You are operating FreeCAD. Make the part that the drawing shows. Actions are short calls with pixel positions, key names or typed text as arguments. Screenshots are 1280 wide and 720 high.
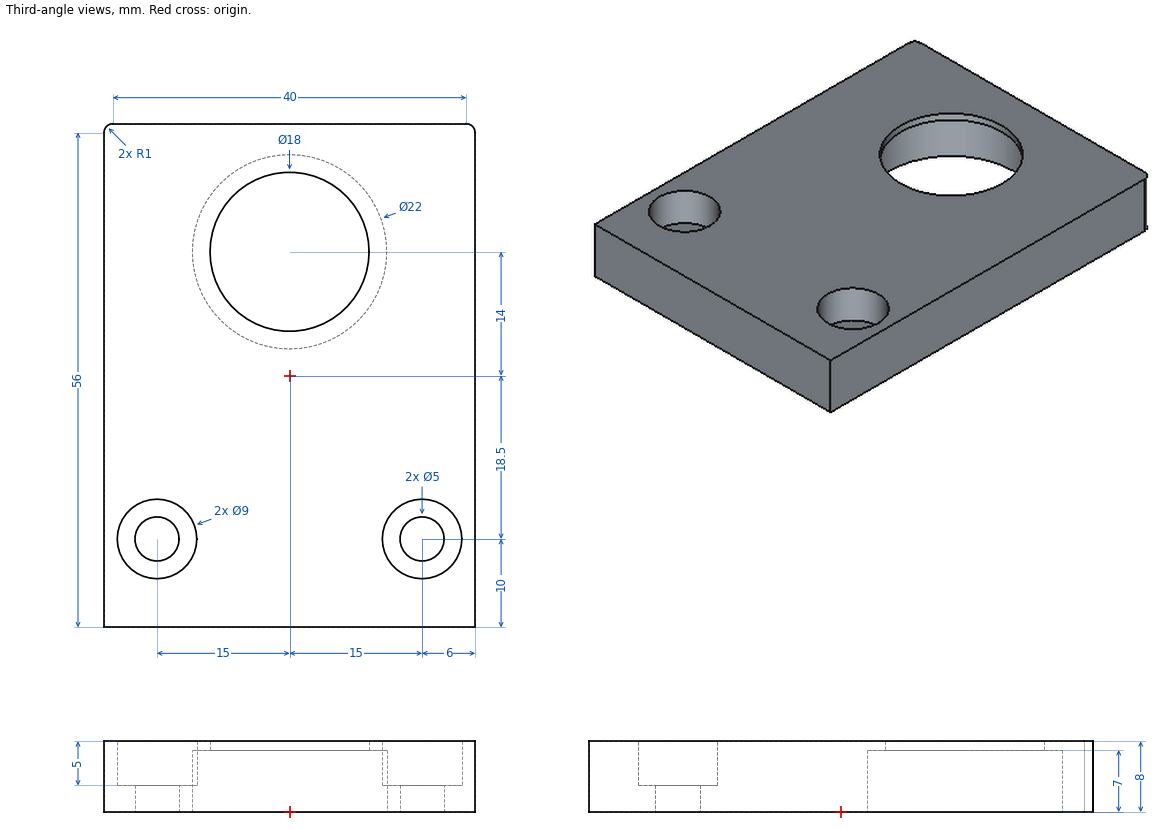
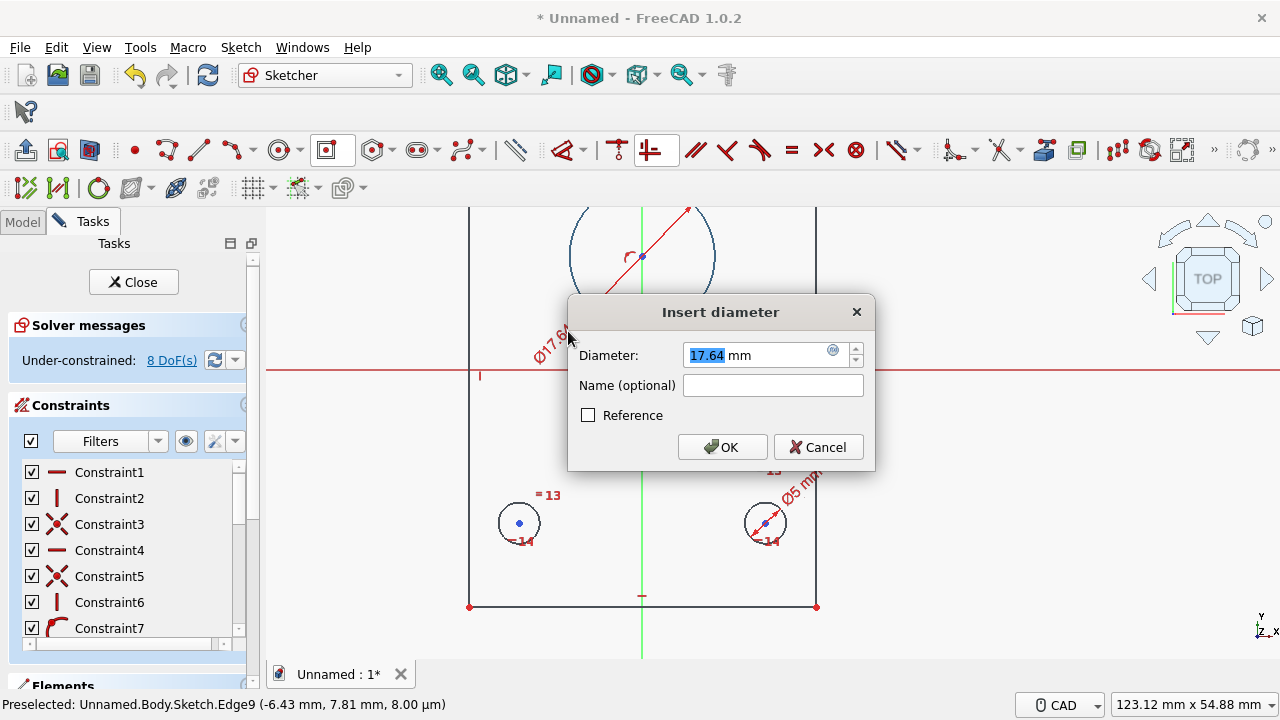
text(18)
key(Return)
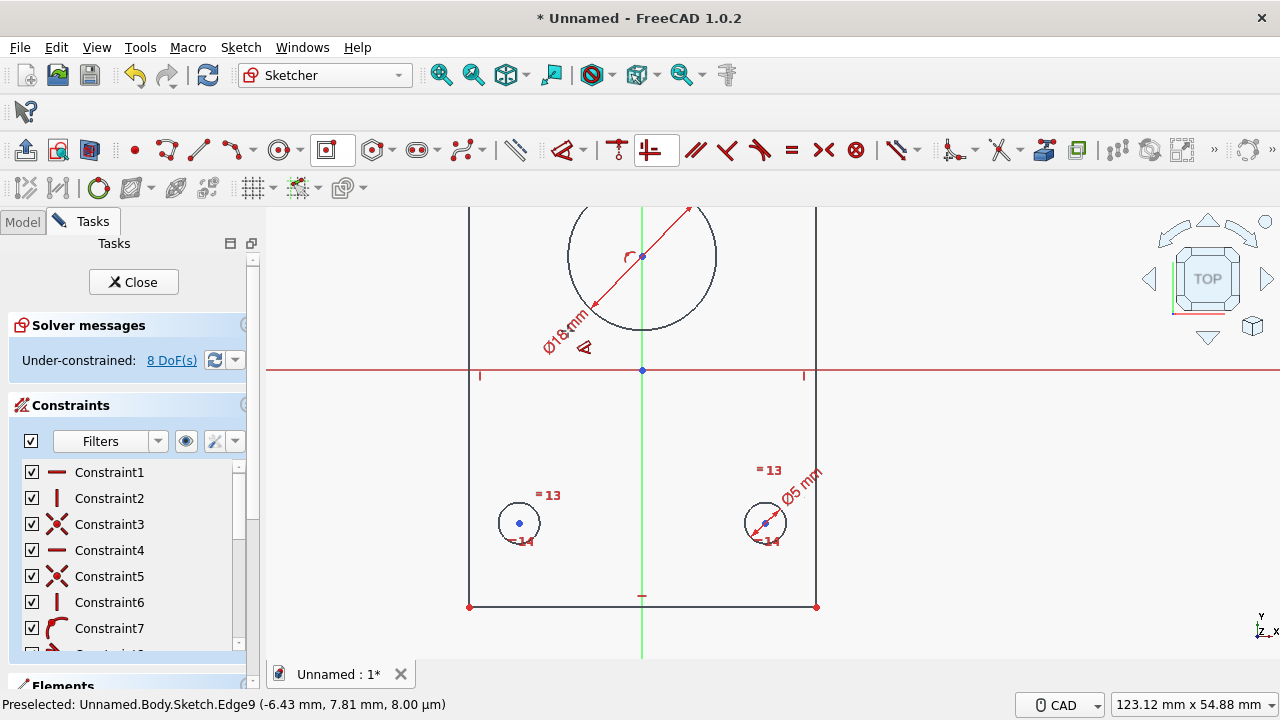
scroll(780, 509, down, 3)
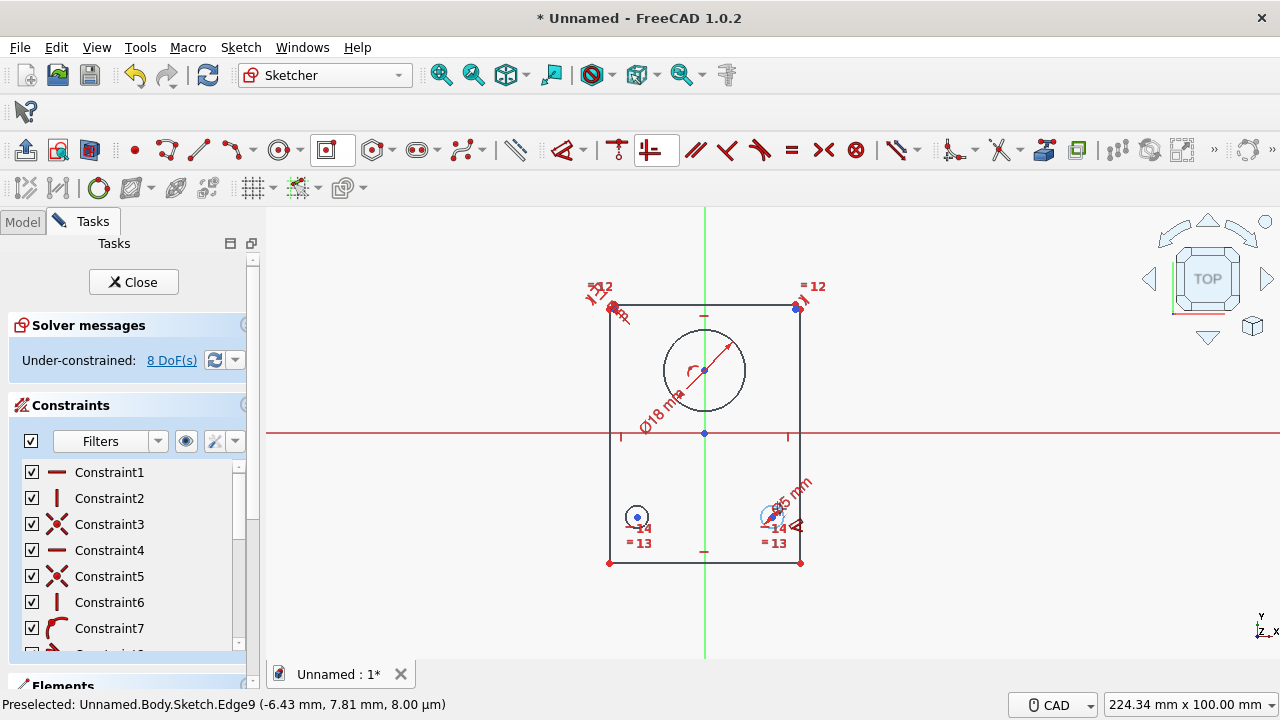
click(741, 305)
click(663, 271)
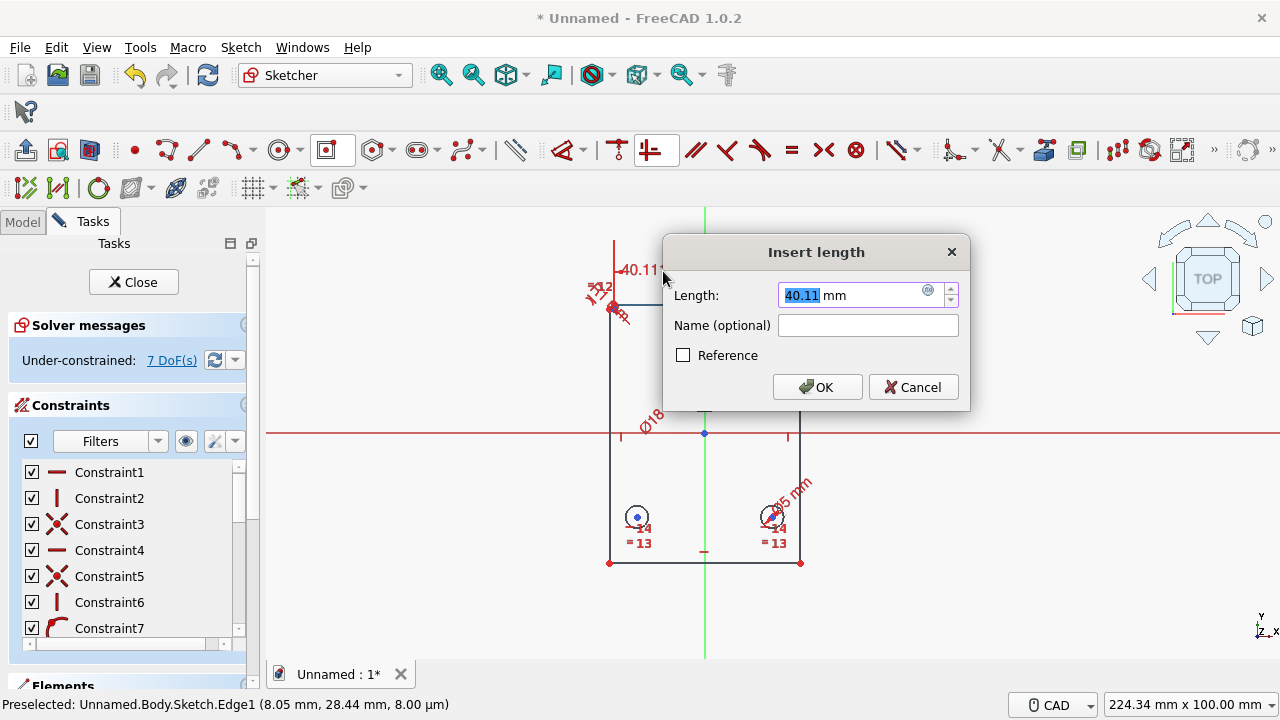
text(40)
key(Return)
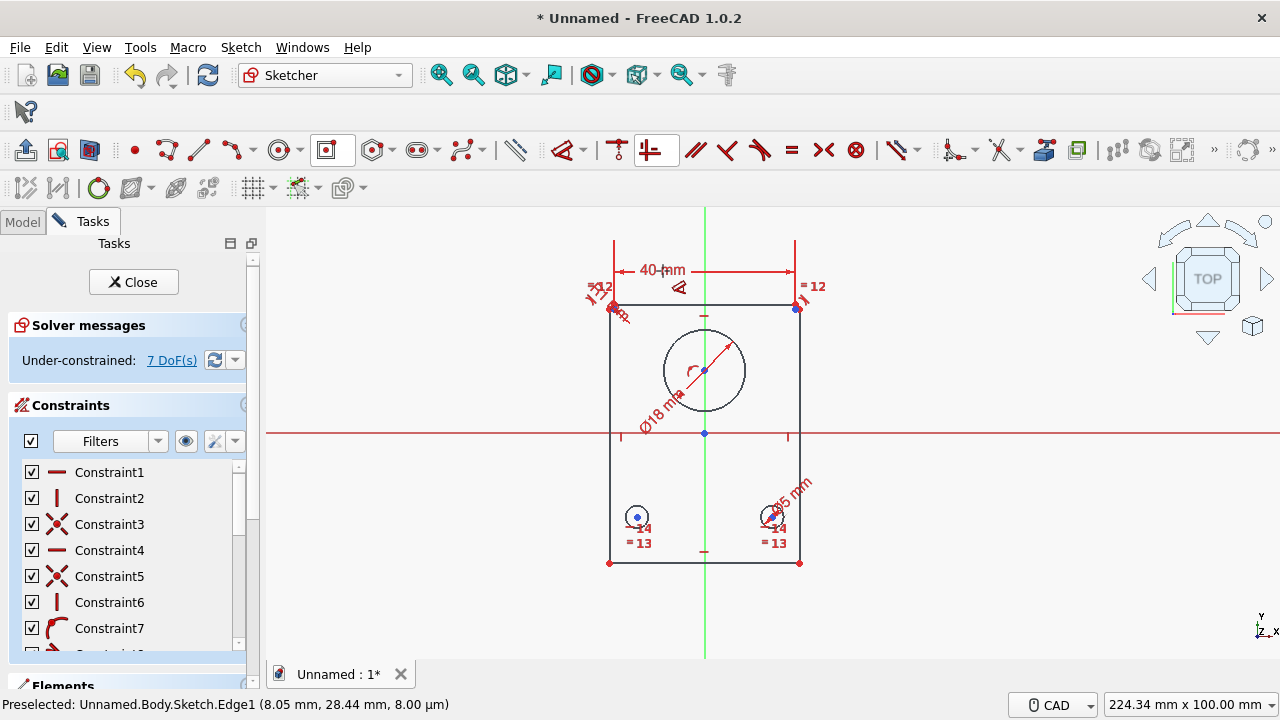
click(610, 385)
click(576, 378)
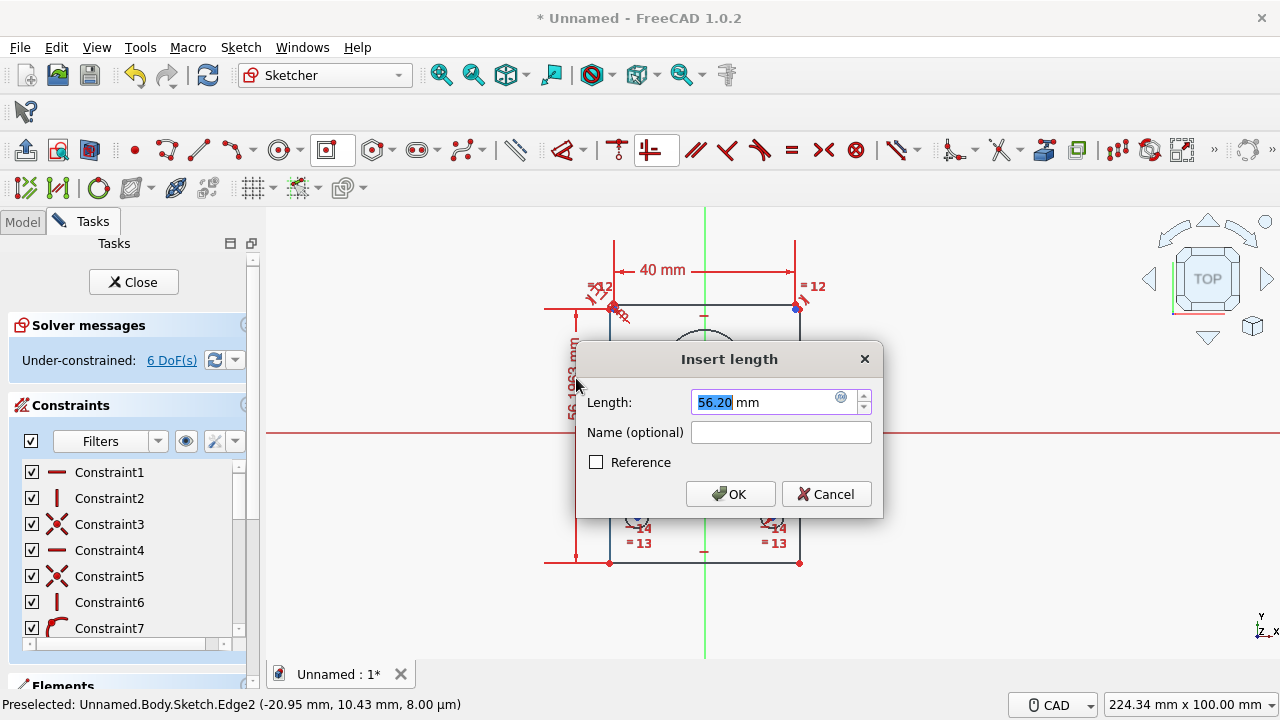
text(56)
key(Return)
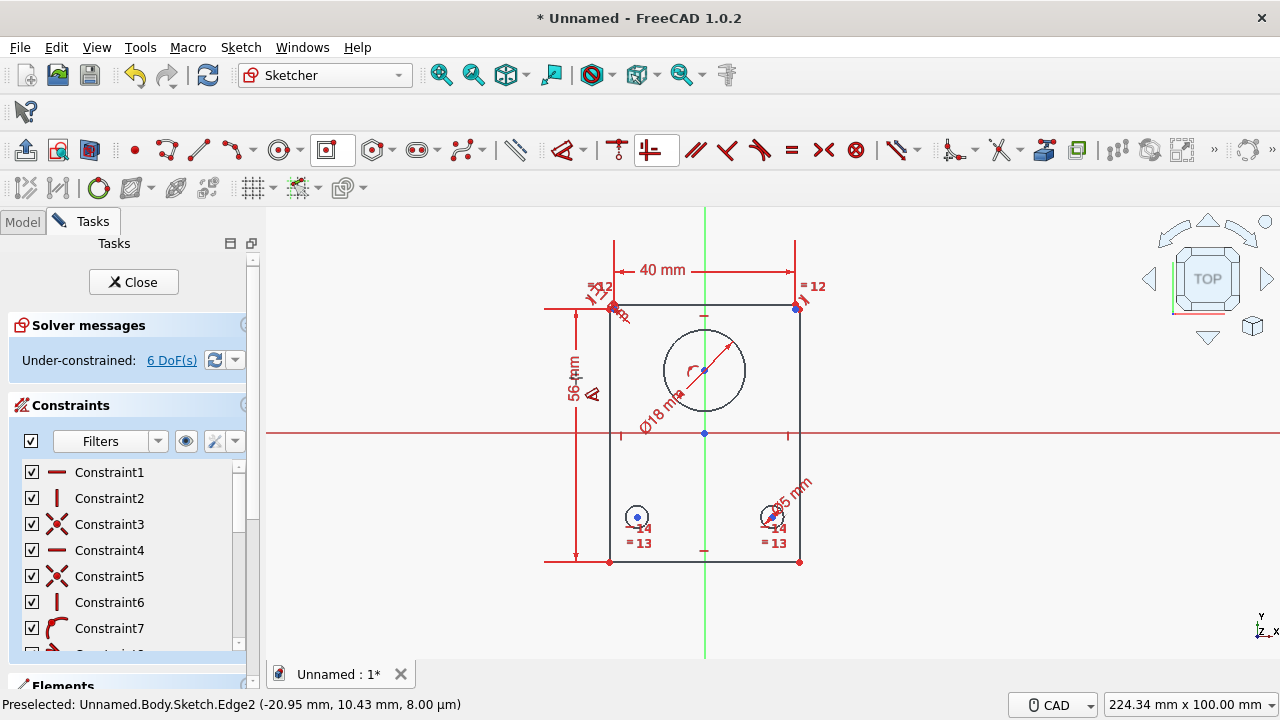
click(772, 517)
click(754, 399)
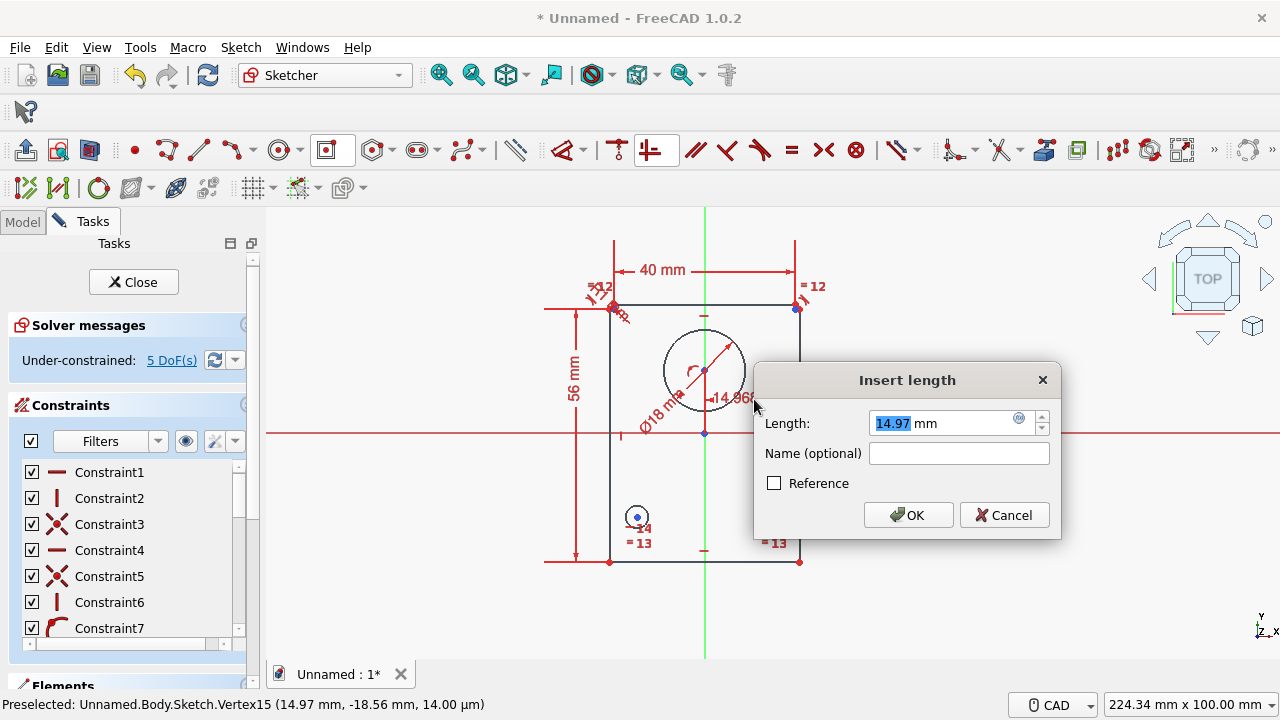
text(15)
key(Return)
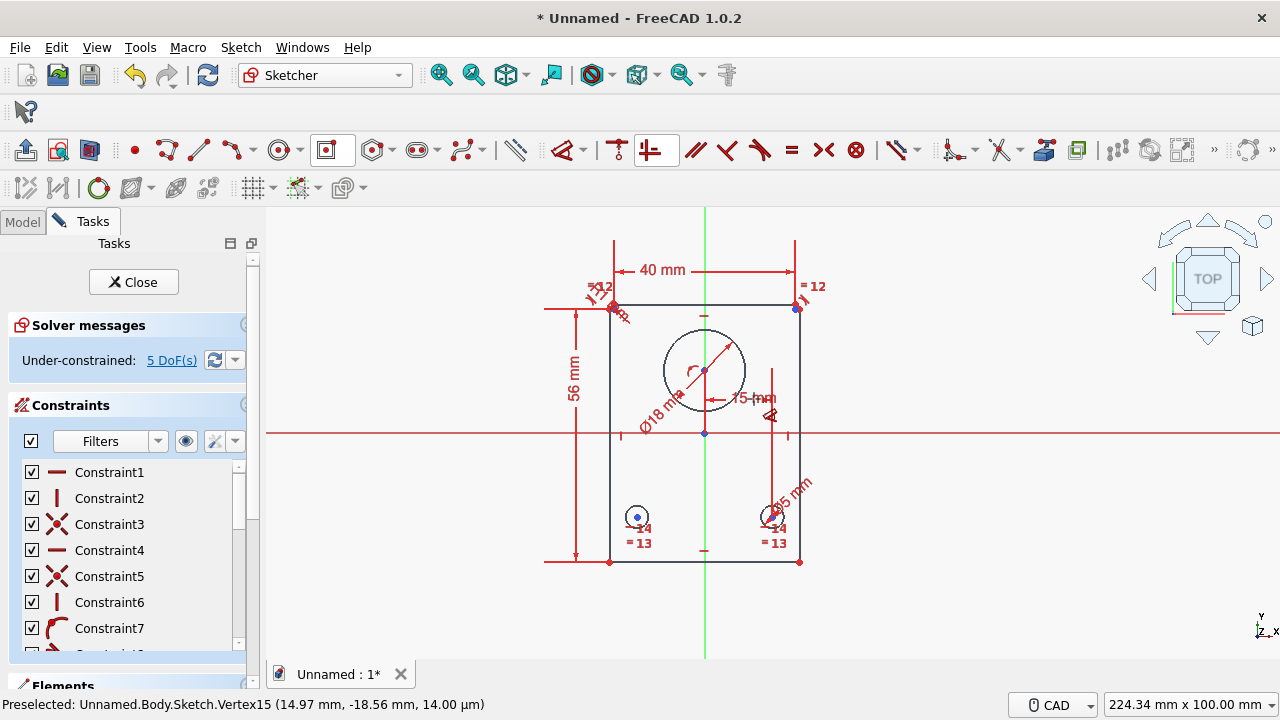
click(637, 517)
click(686, 375)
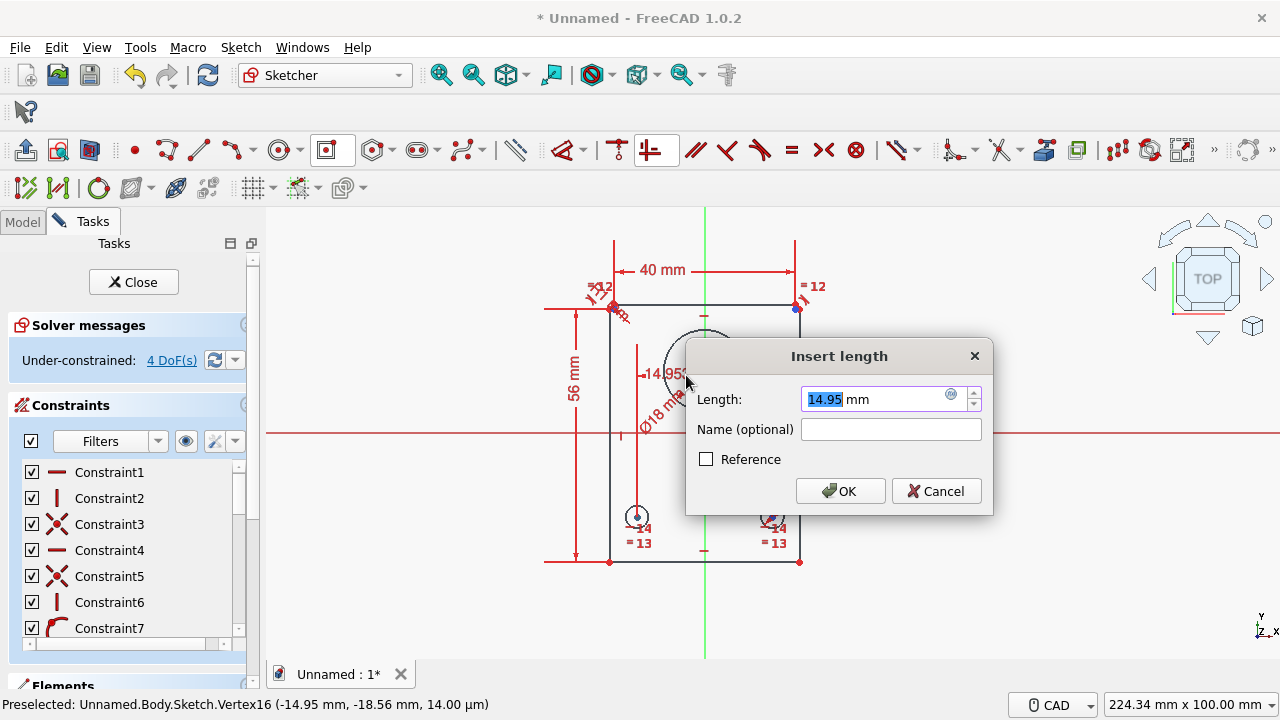
text(15)
key(Return)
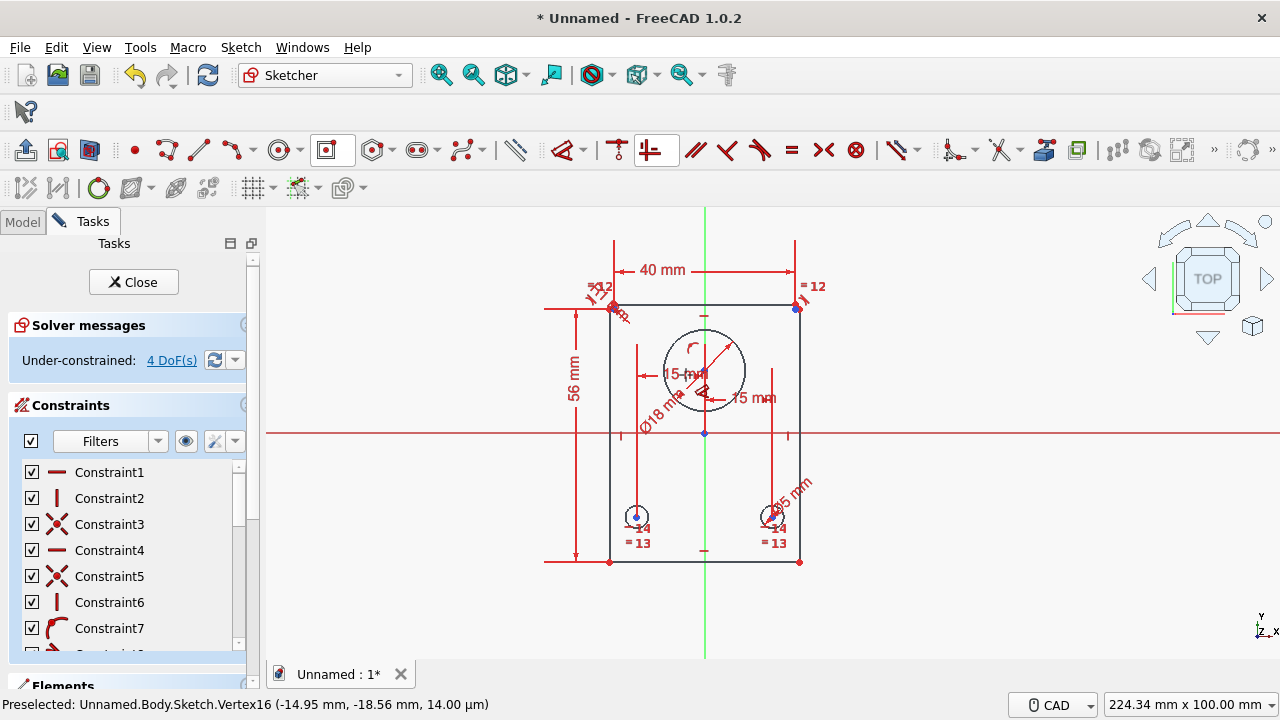
click(705, 371)
click(835, 402)